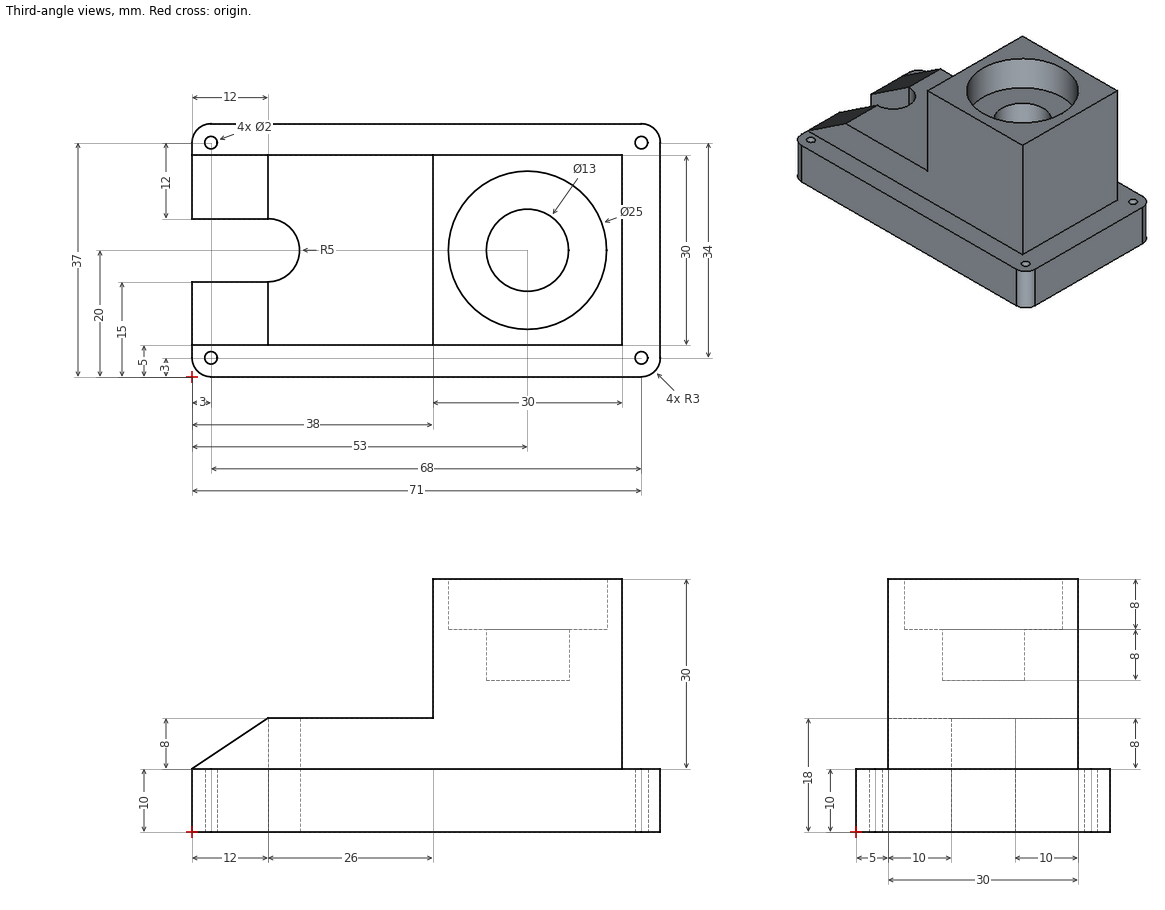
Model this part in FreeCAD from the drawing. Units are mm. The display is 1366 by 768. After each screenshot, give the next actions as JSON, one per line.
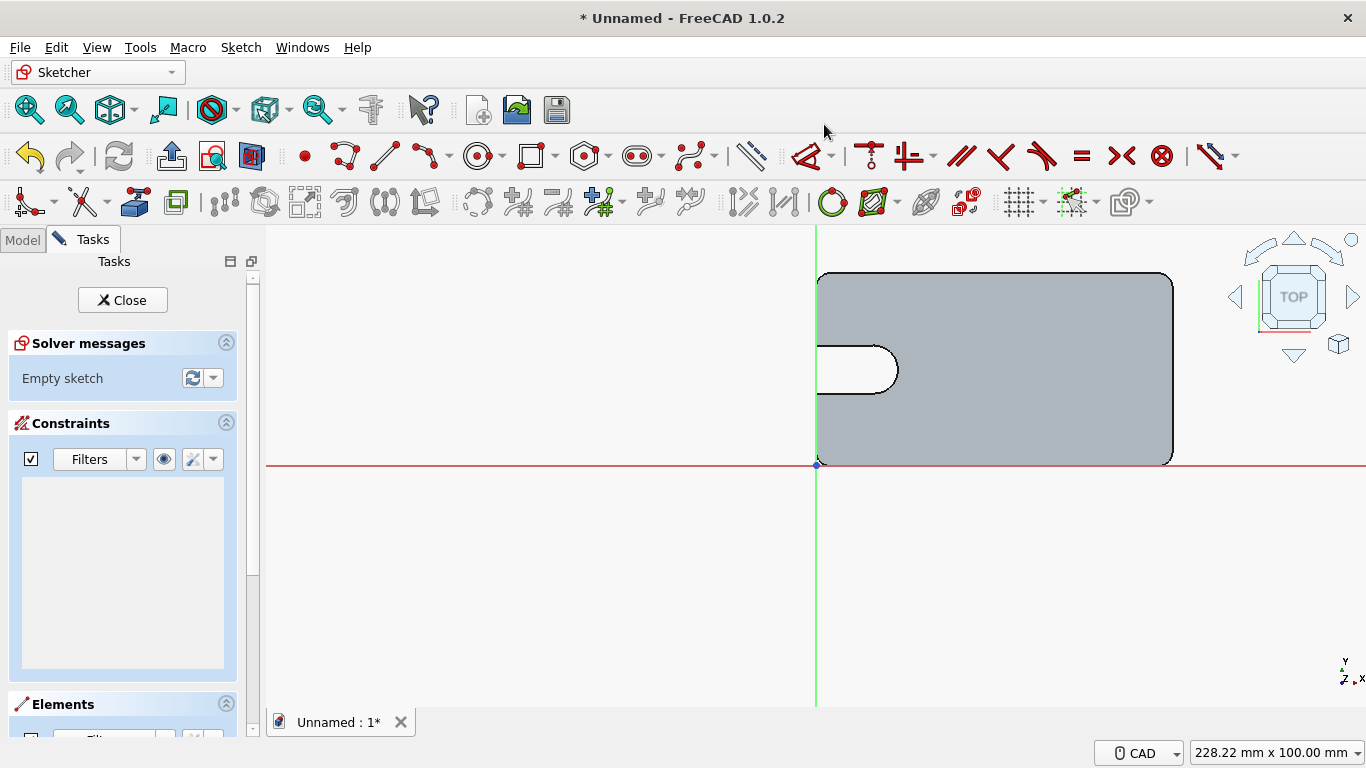
{"action": "scroll", "coordinate": [1201, 279], "scroll_direction": "up", "scroll_amount": 3}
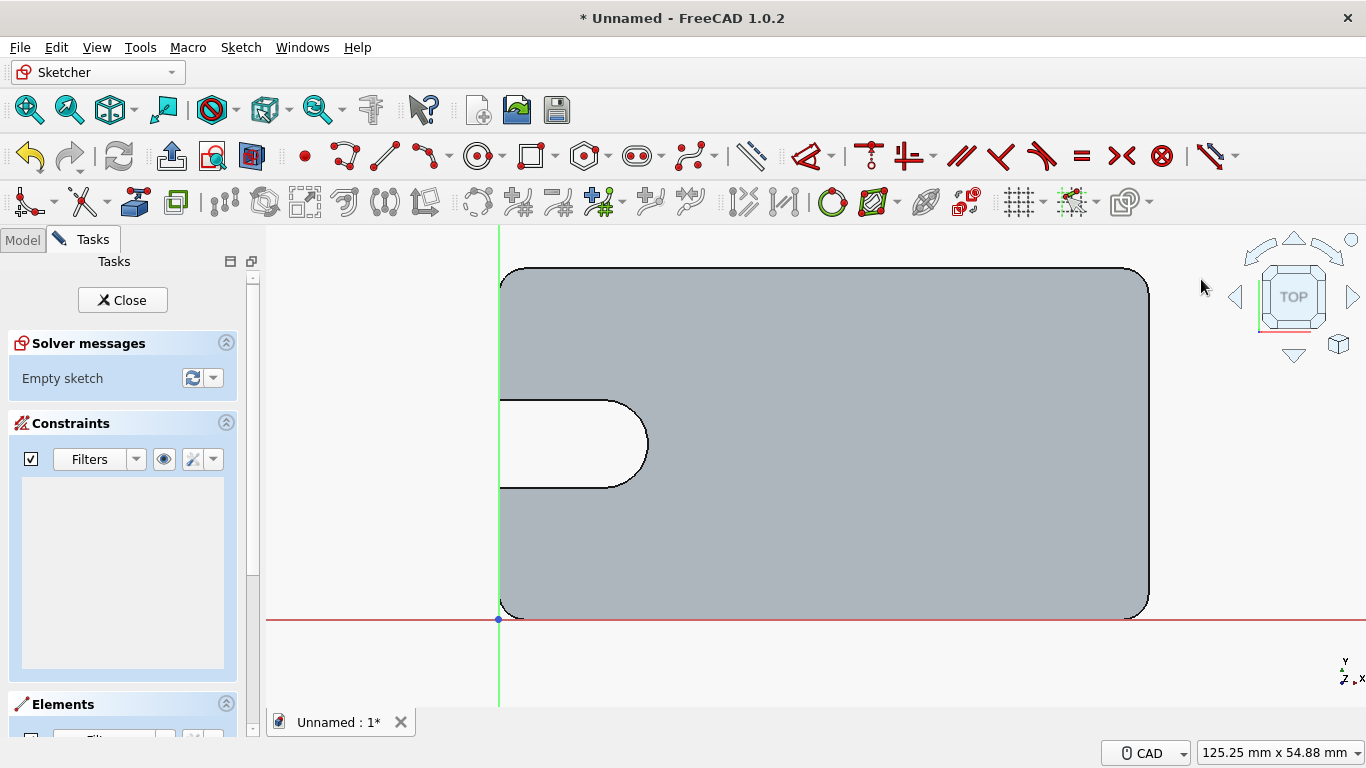
{"action": "left_click", "coordinate": [532, 156]}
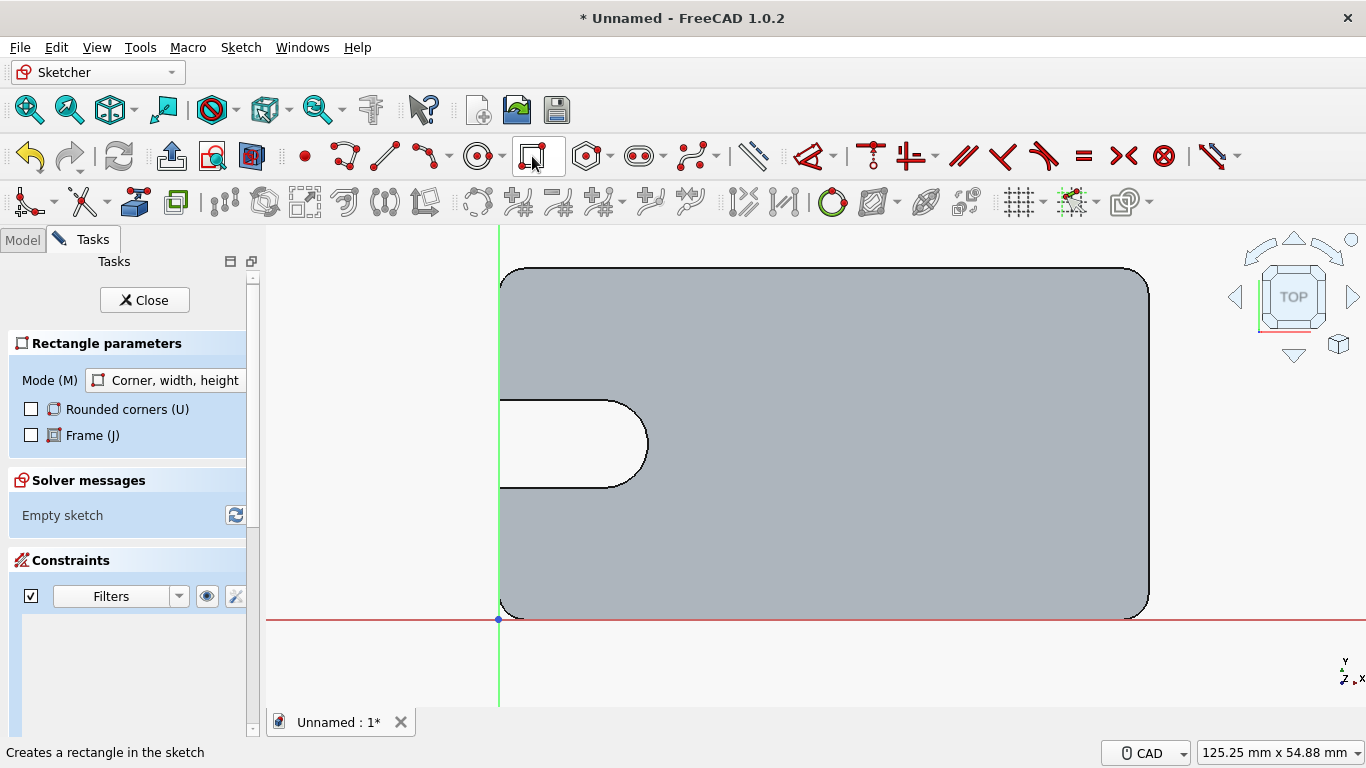
{"action": "left_click", "coordinate": [833, 312]}
{"action": "left_click", "coordinate": [1096, 576]}
{"action": "key", "text": "Escape"}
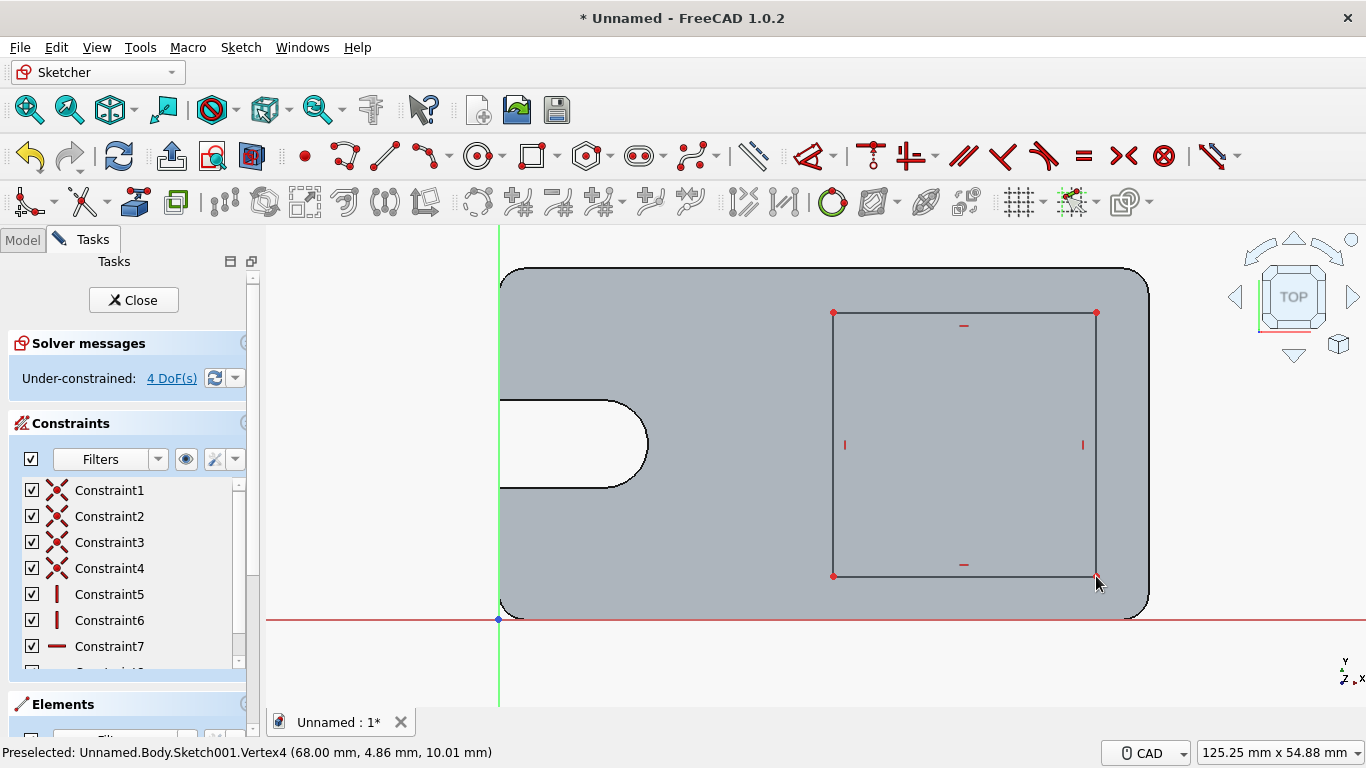
{"action": "left_click", "coordinate": [808, 156]}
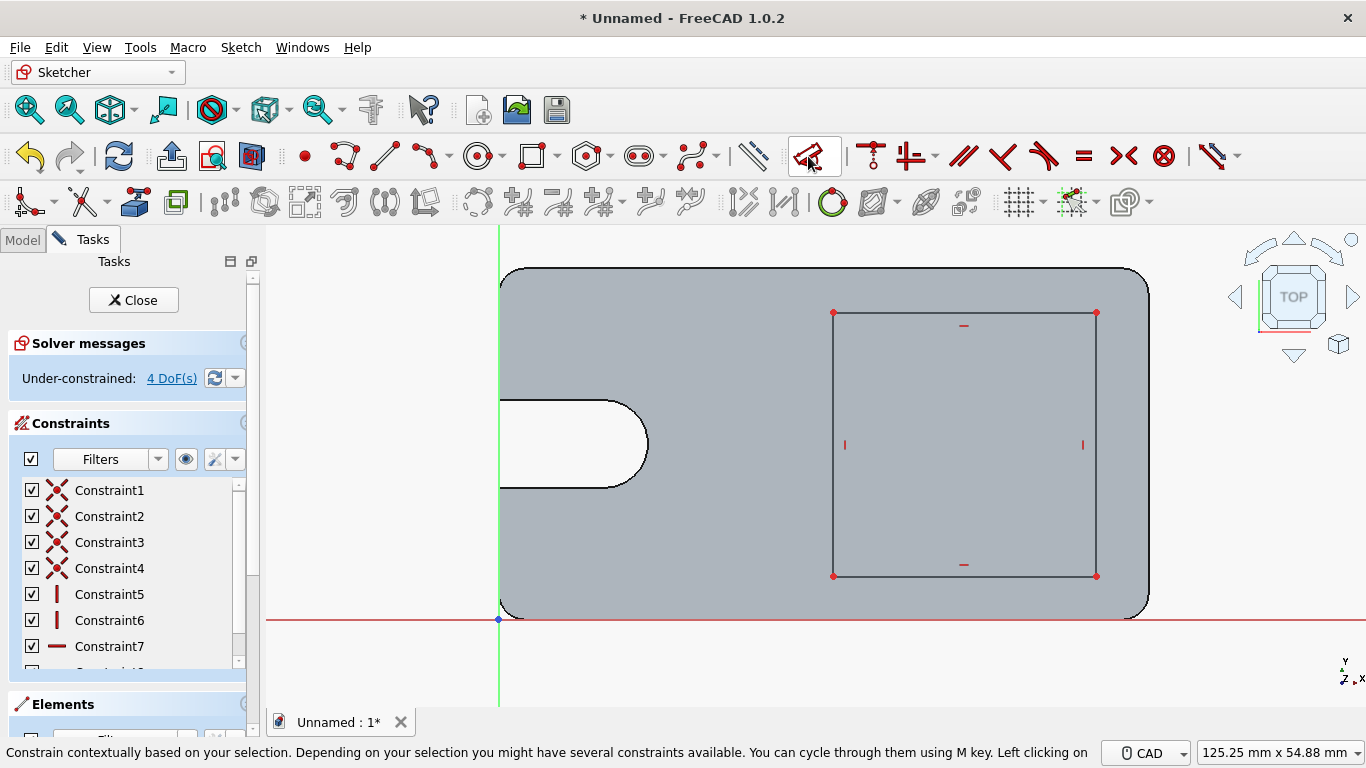
{"action": "left_click", "coordinate": [833, 392]}
{"action": "left_click", "coordinate": [867, 445]}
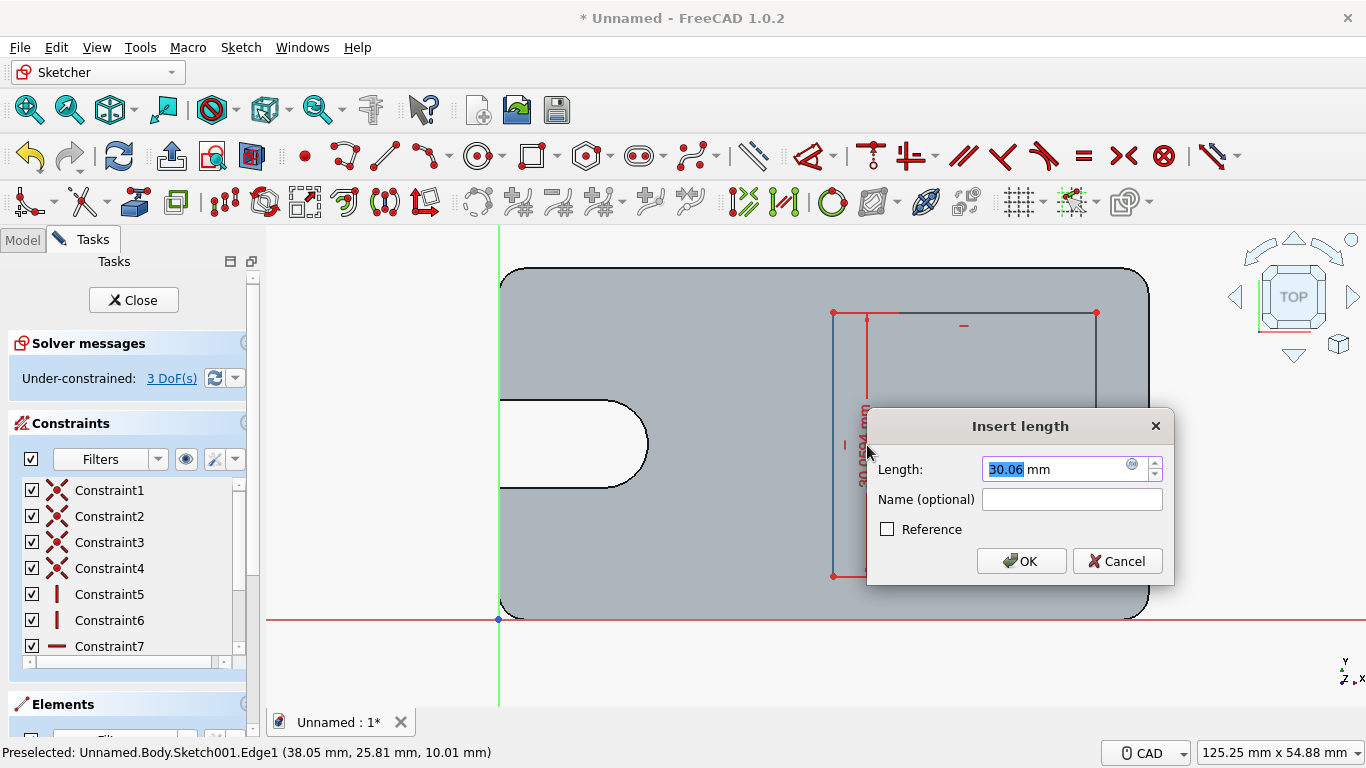
{"action": "type", "text": "30"}
{"action": "key", "text": "Return"}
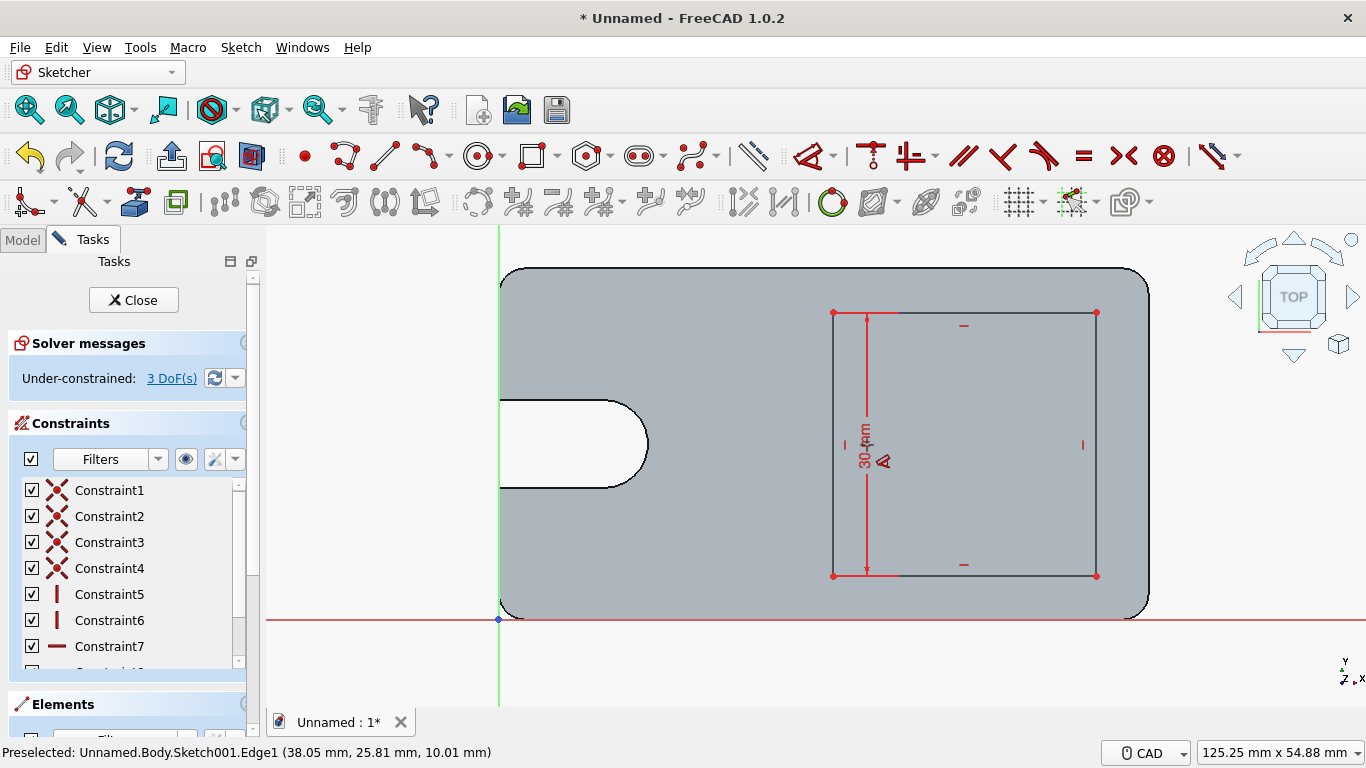
{"action": "left_click", "coordinate": [912, 576]}
{"action": "left_click", "coordinate": [964, 542]}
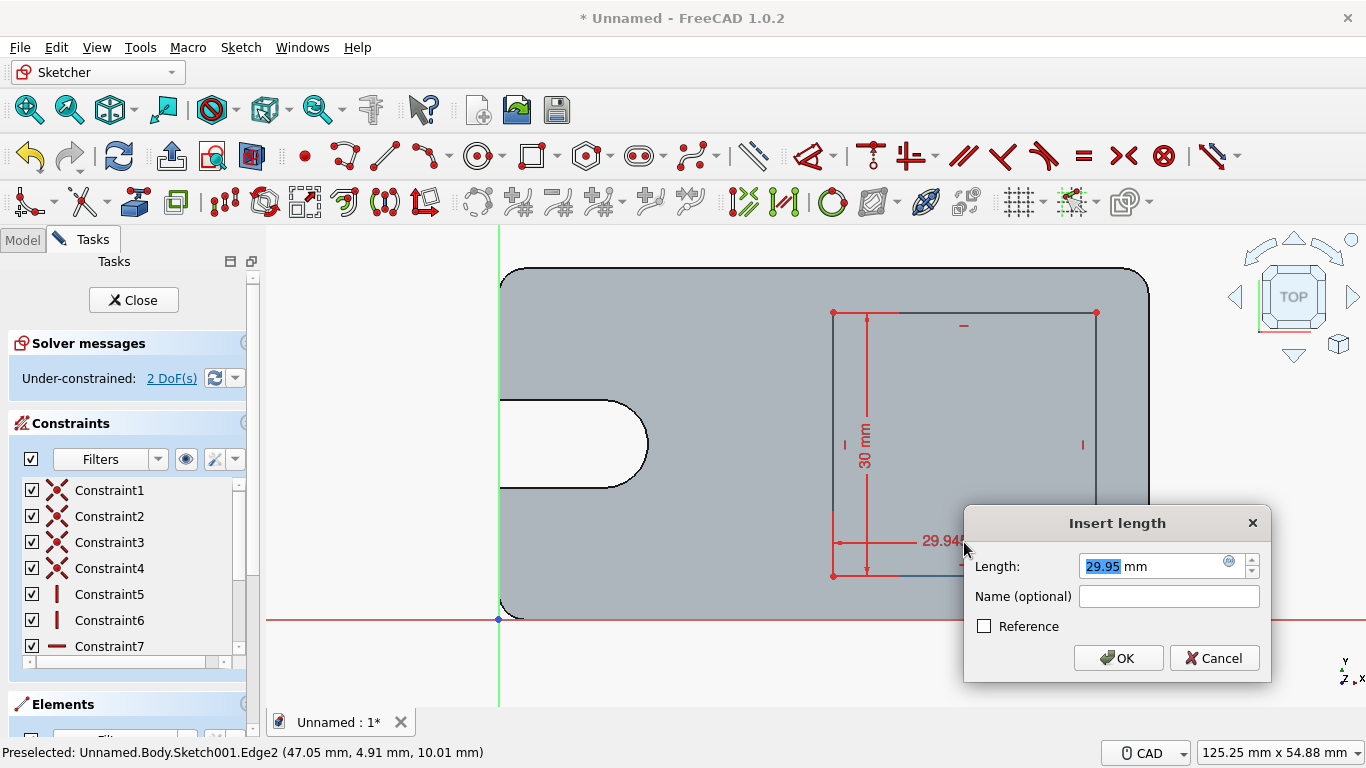
{"action": "type", "text": "30"}
{"action": "key", "text": "Return"}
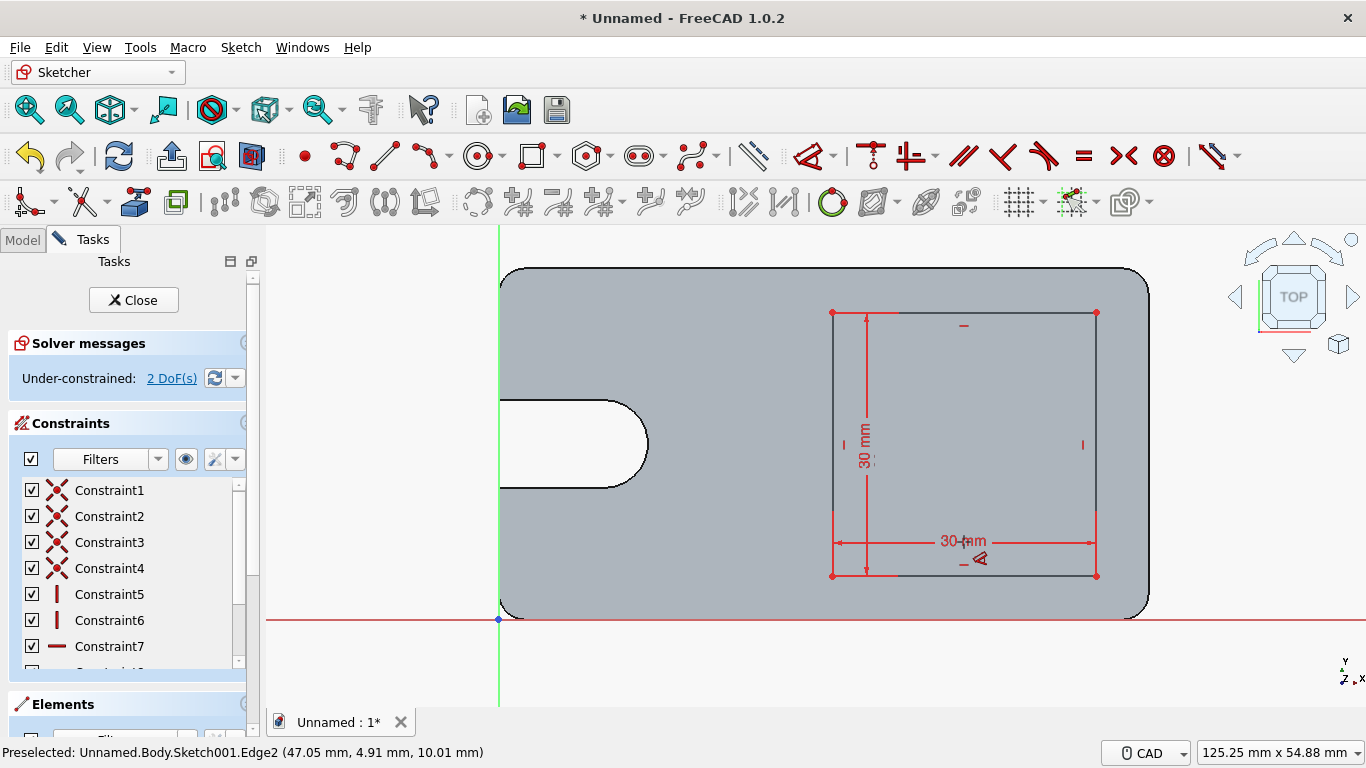
{"action": "left_click", "coordinate": [833, 576]}
{"action": "left_click", "coordinate": [465, 598]}